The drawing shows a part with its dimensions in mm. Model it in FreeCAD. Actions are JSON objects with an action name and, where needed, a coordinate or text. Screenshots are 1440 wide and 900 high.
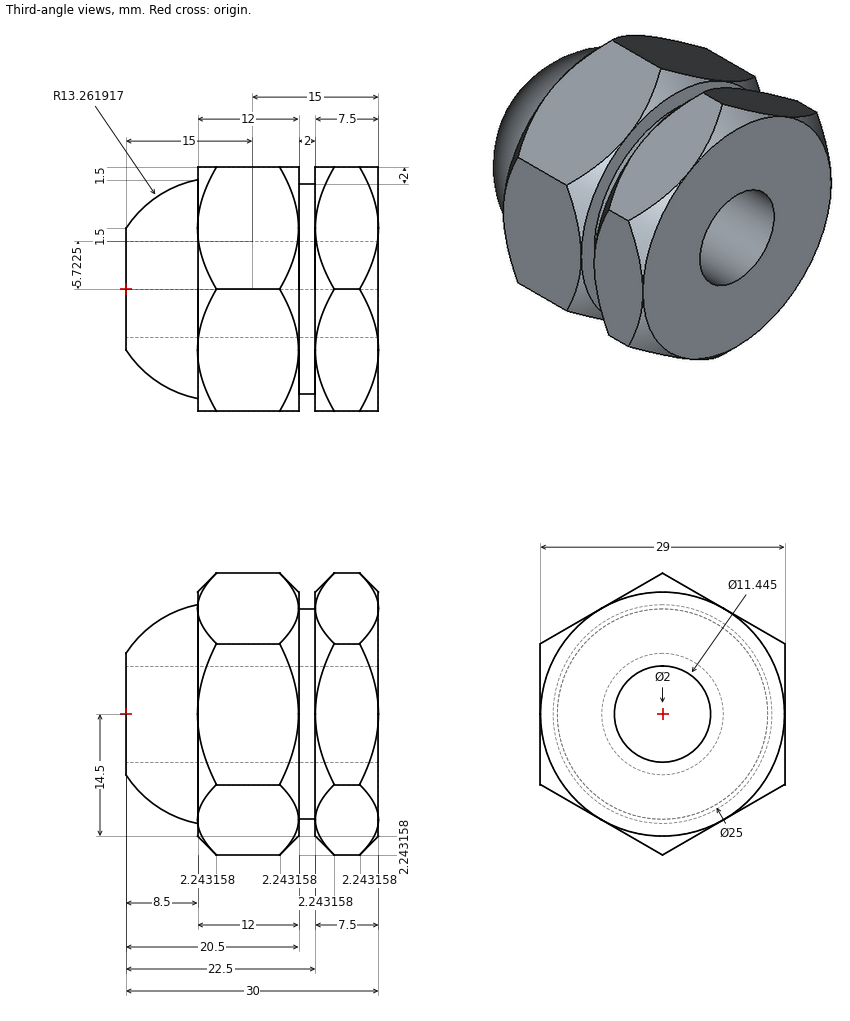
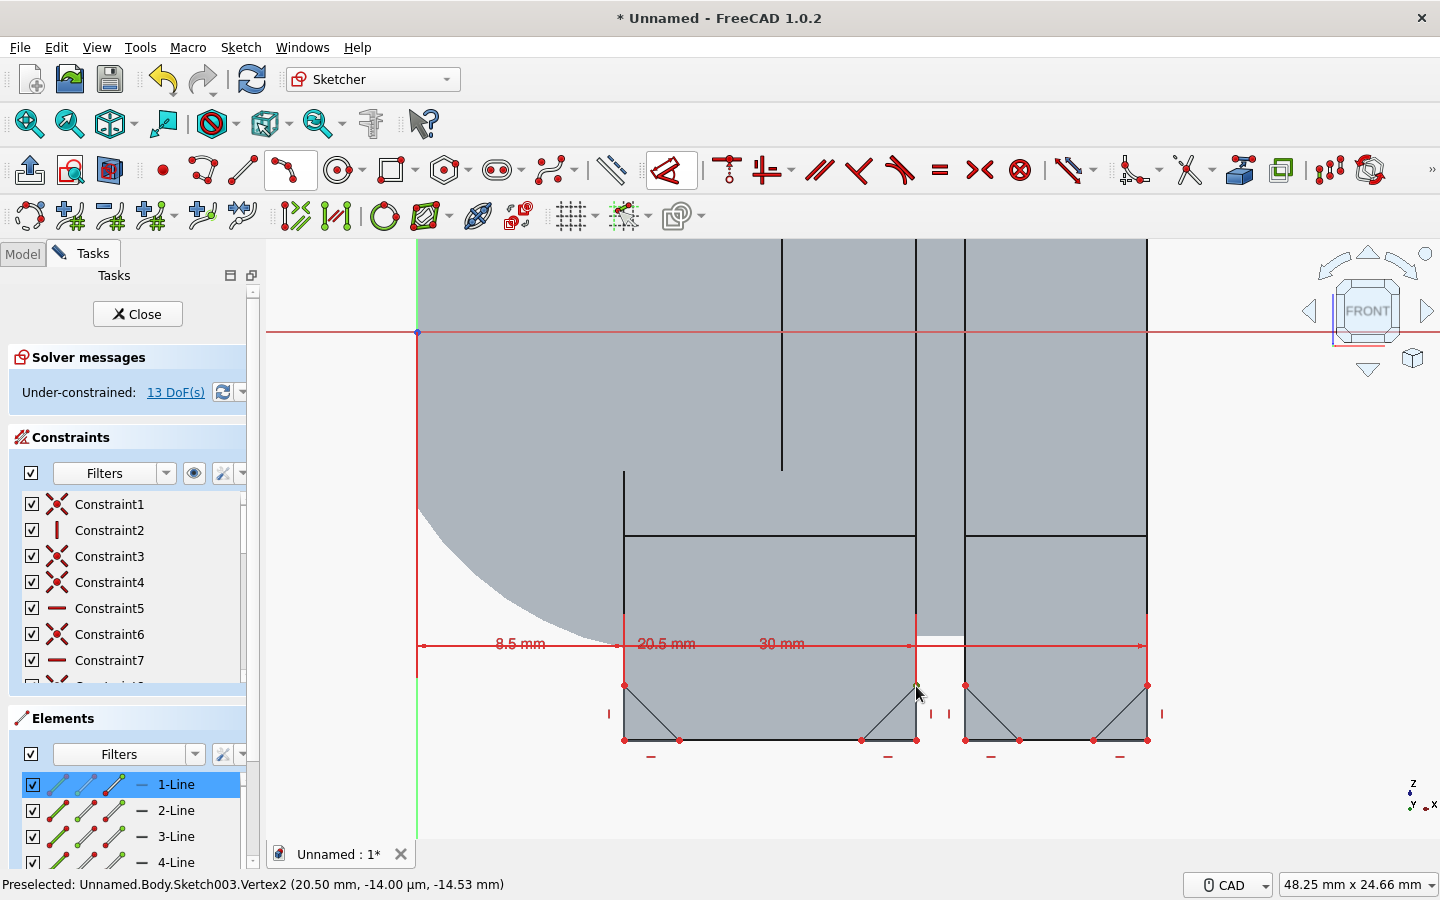
{"action": "key", "text": "i"}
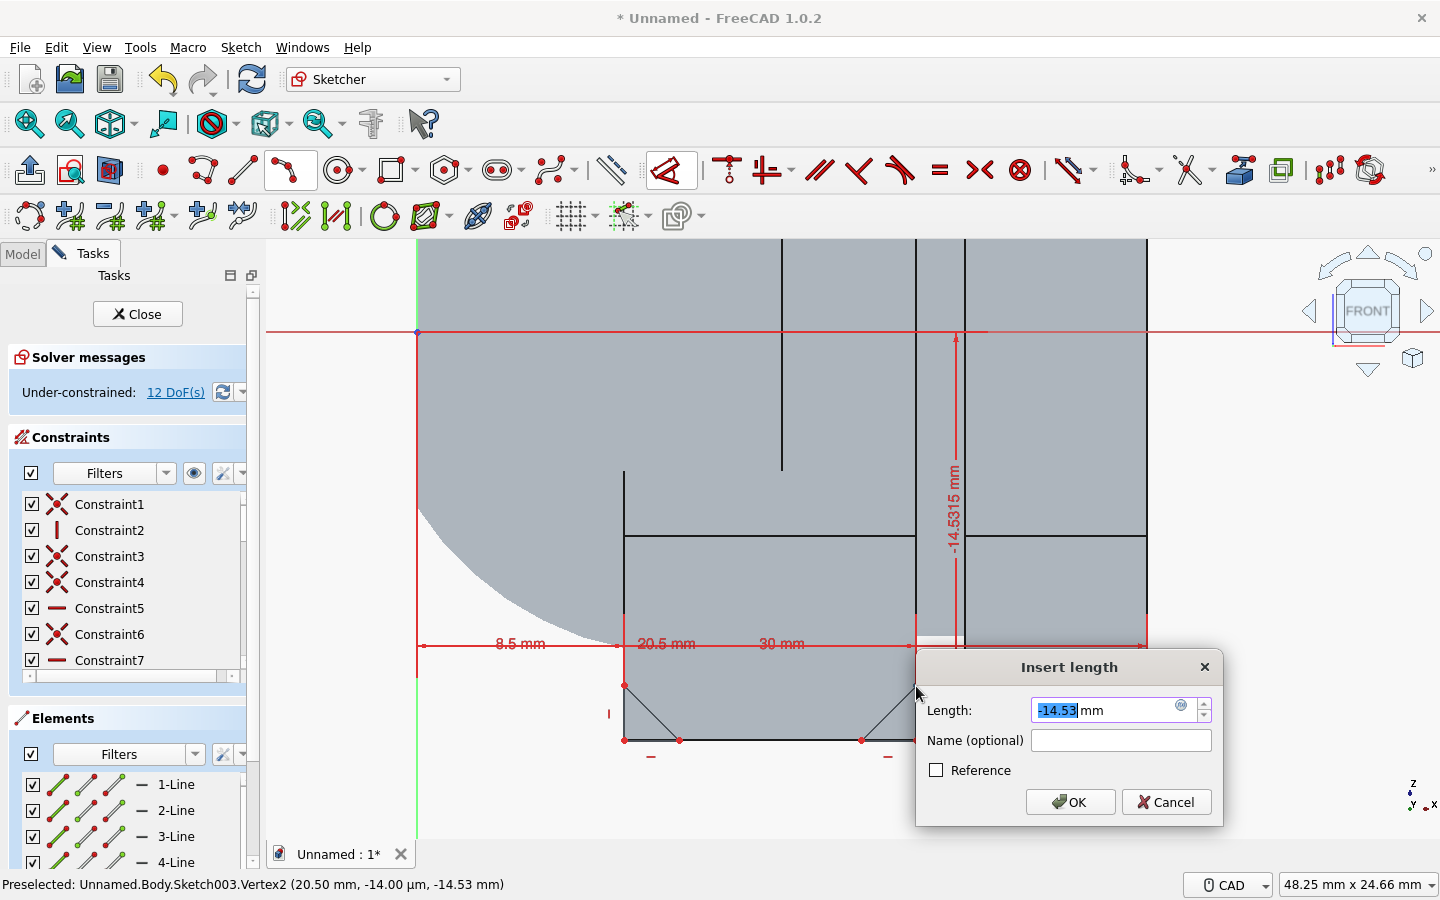
{"action": "type", "text": "-14.5"}
{"action": "key", "text": "Return"}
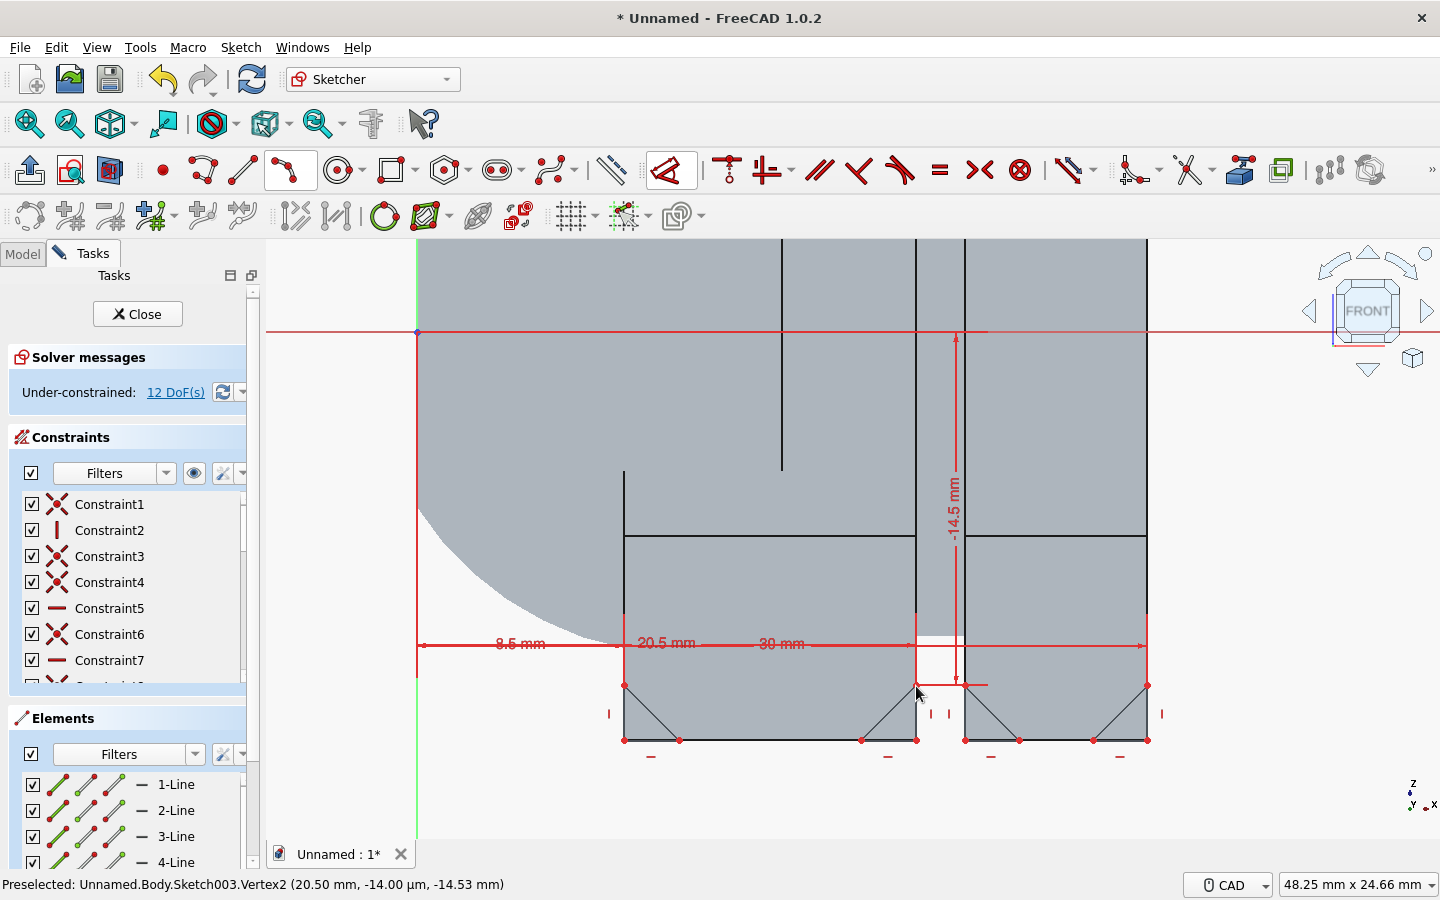
{"action": "left_click", "coordinate": [965, 686]}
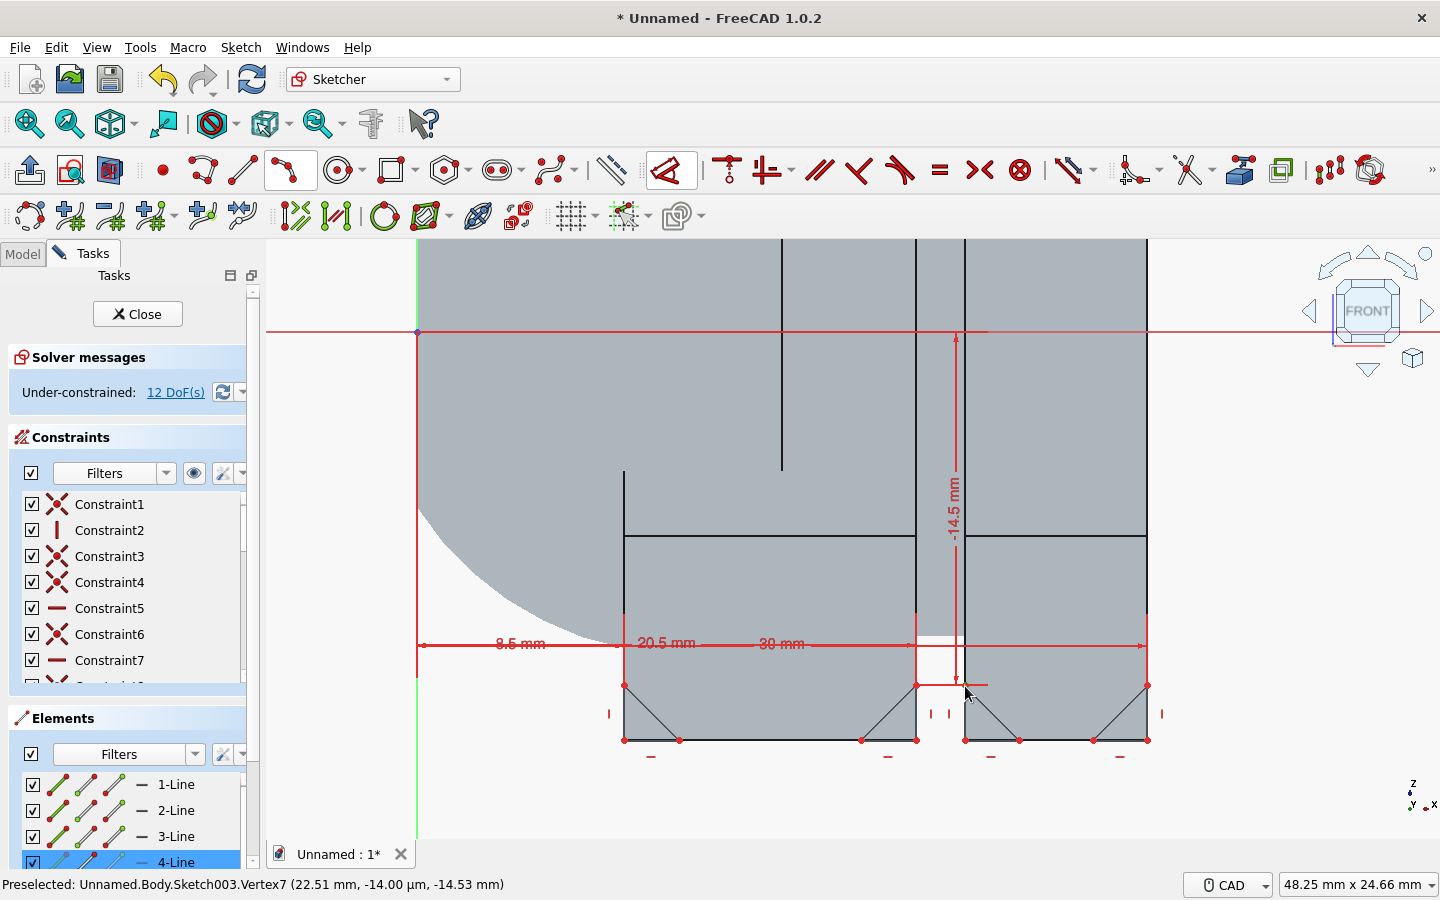
{"action": "key", "text": "l"}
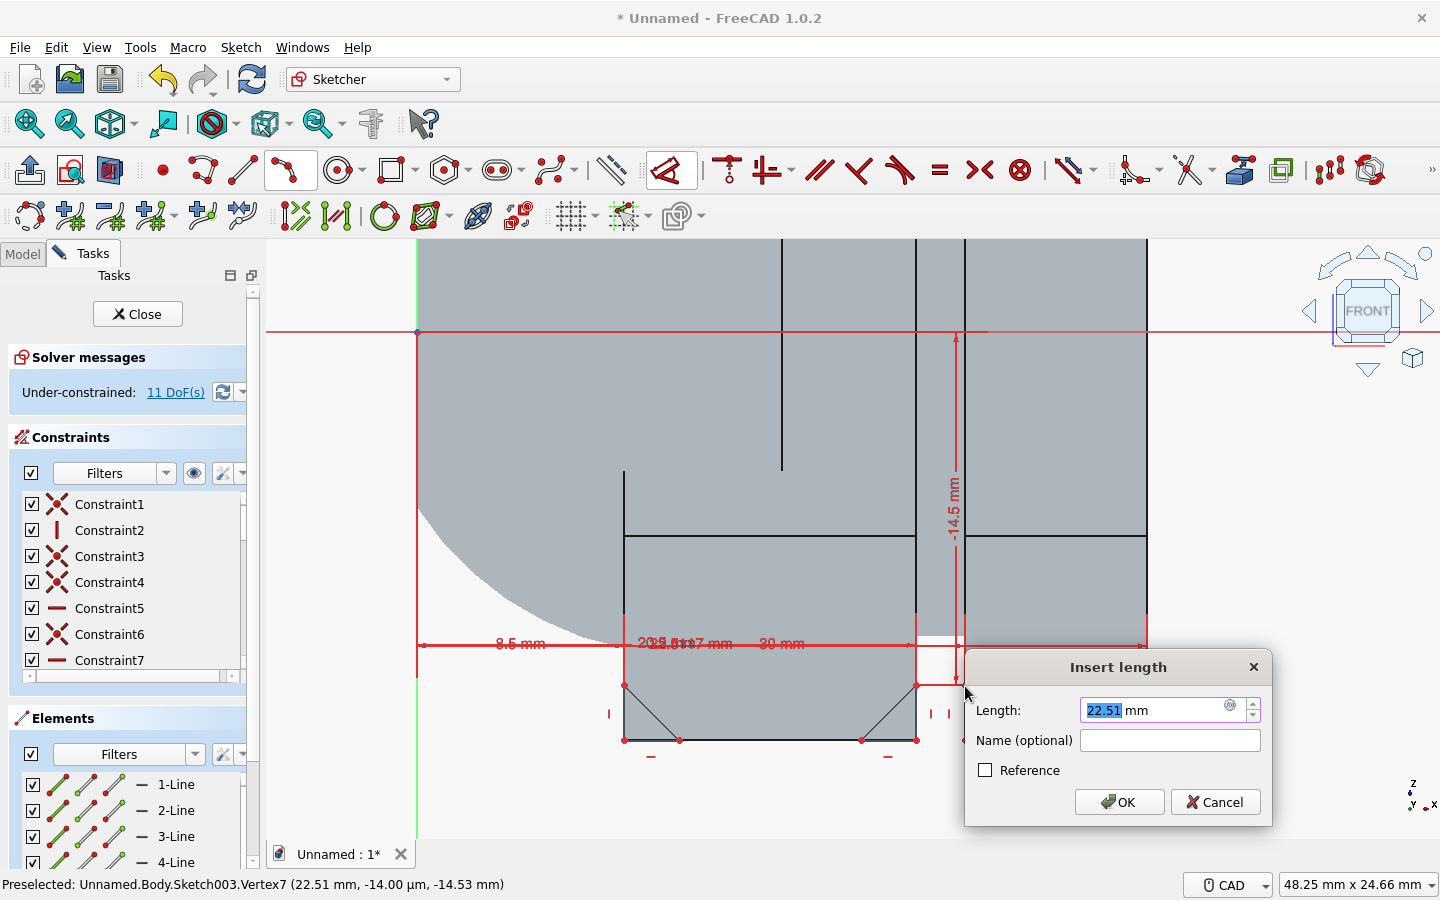
{"action": "type", "text": "22.5"}
{"action": "key", "text": "Return"}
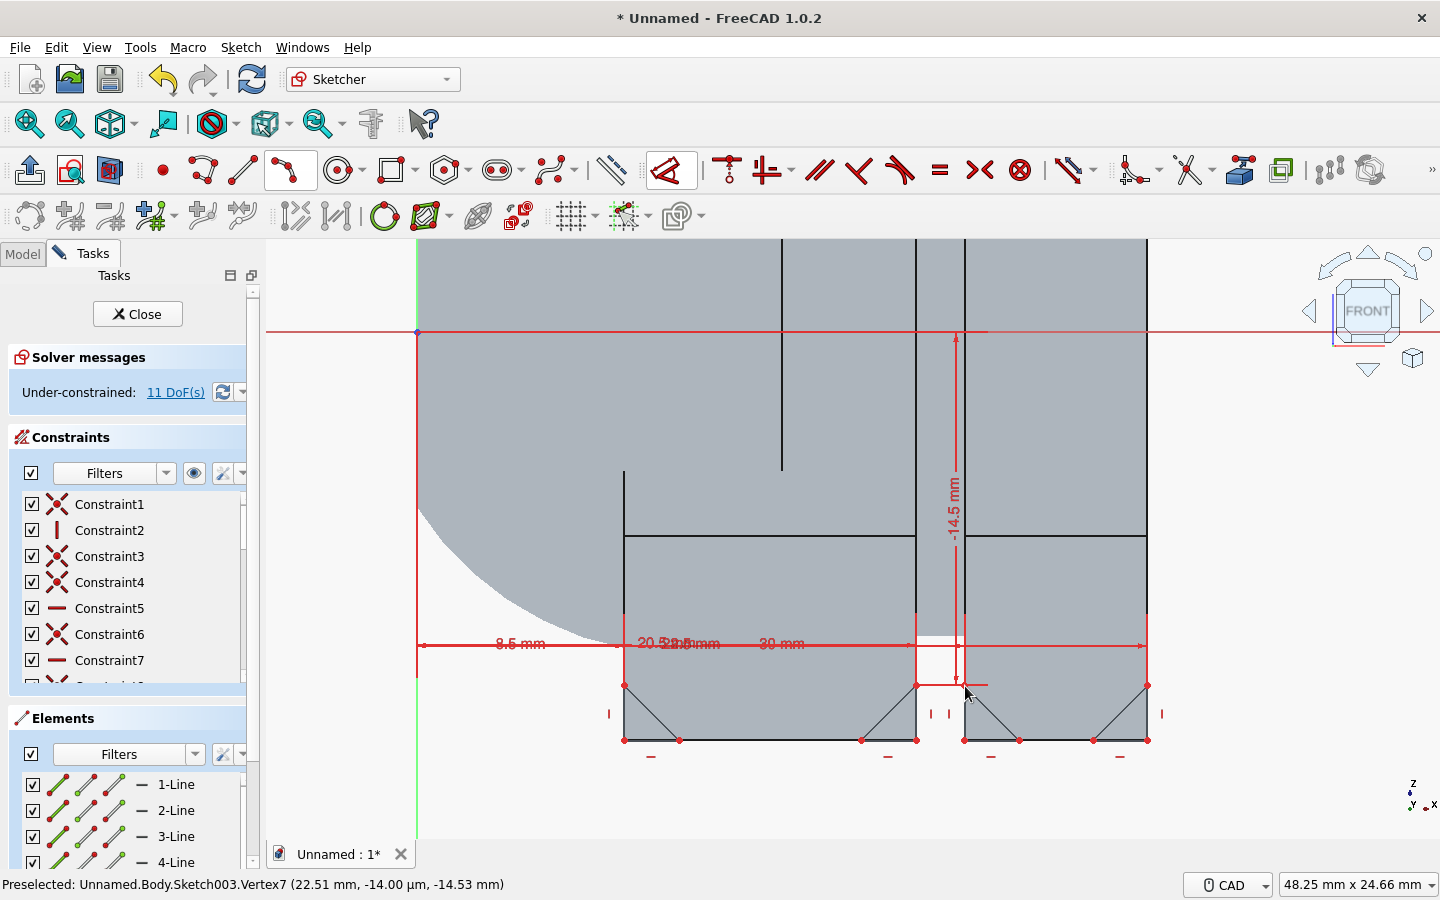
{"action": "left_click", "coordinate": [965, 686]}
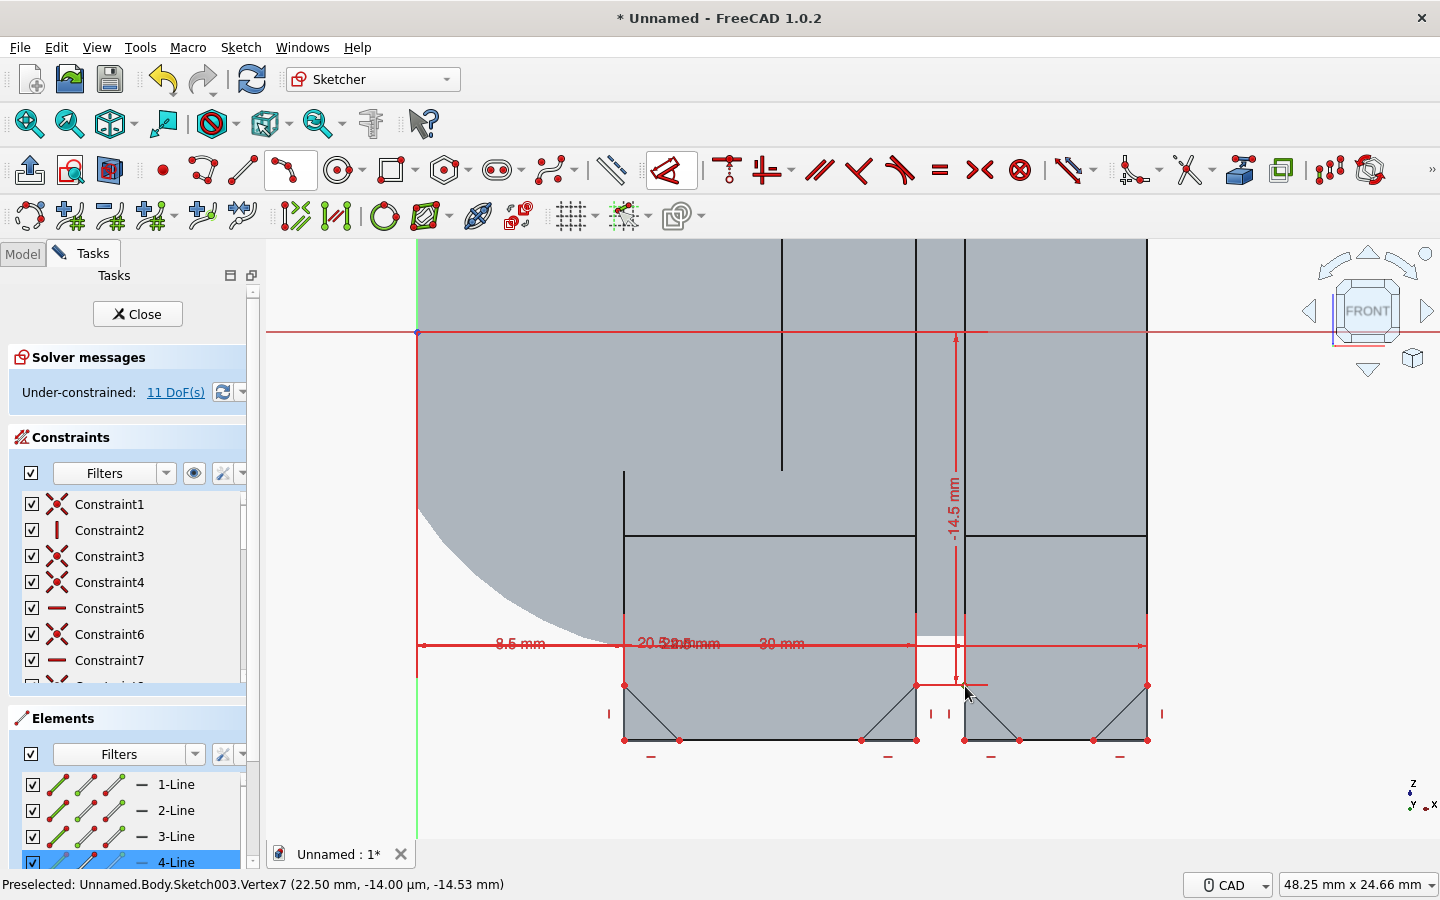
{"action": "key", "text": "i"}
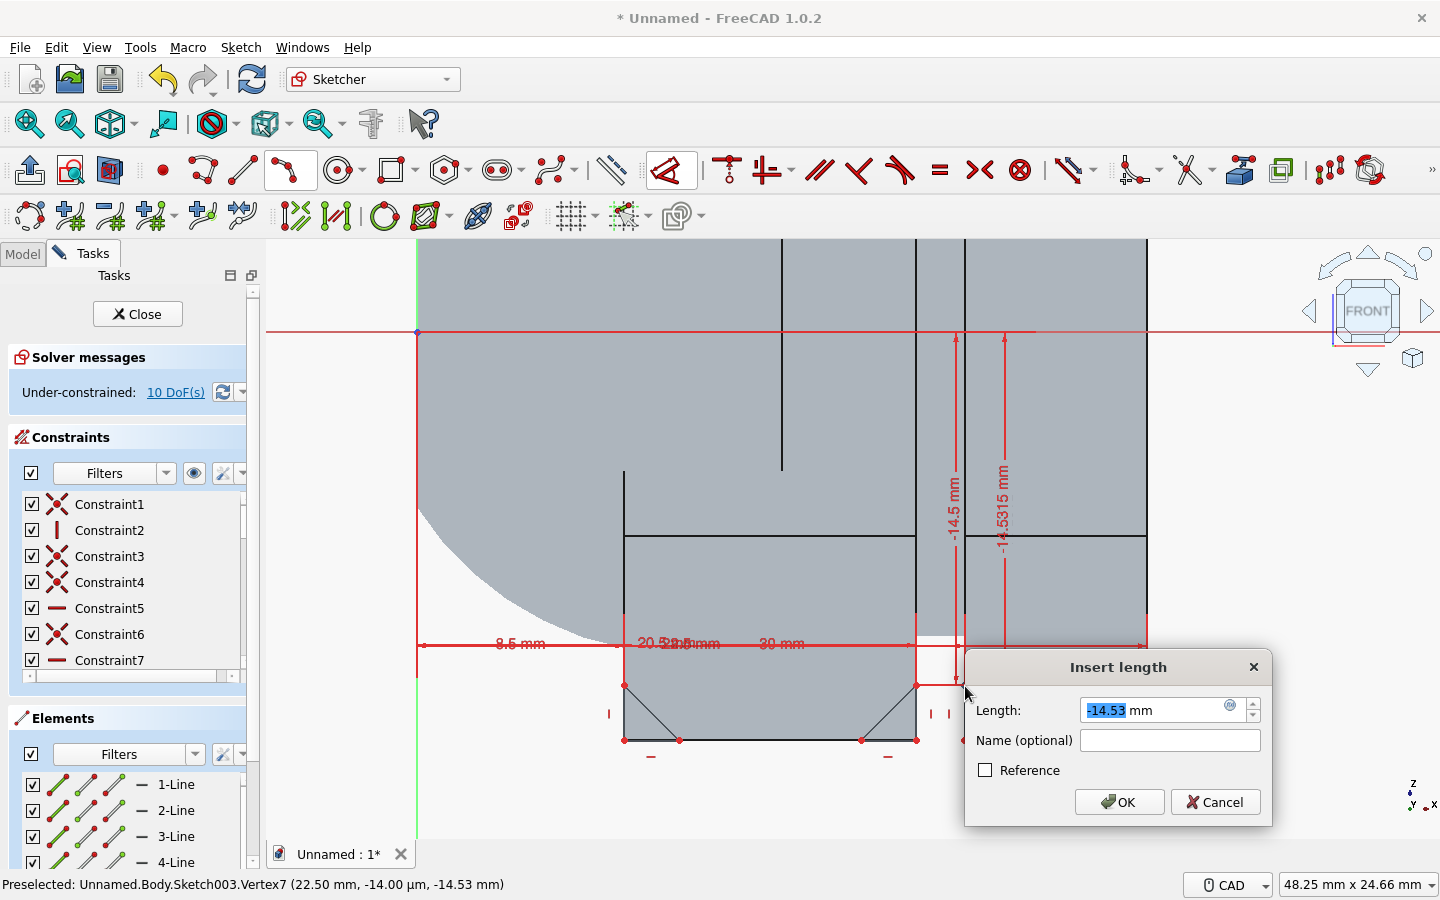
{"action": "type", "text": "-14.5"}
{"action": "key", "text": "Return"}